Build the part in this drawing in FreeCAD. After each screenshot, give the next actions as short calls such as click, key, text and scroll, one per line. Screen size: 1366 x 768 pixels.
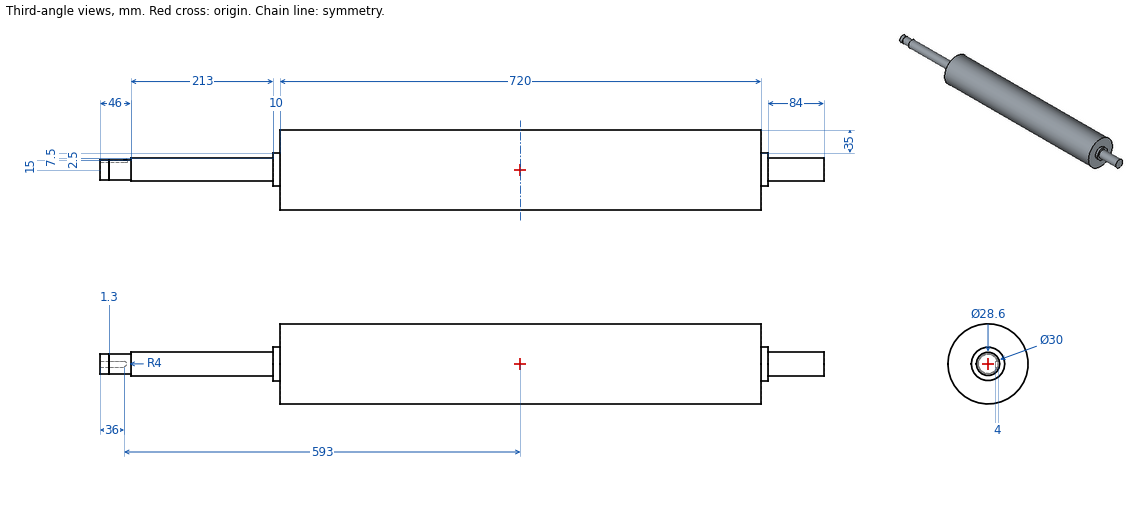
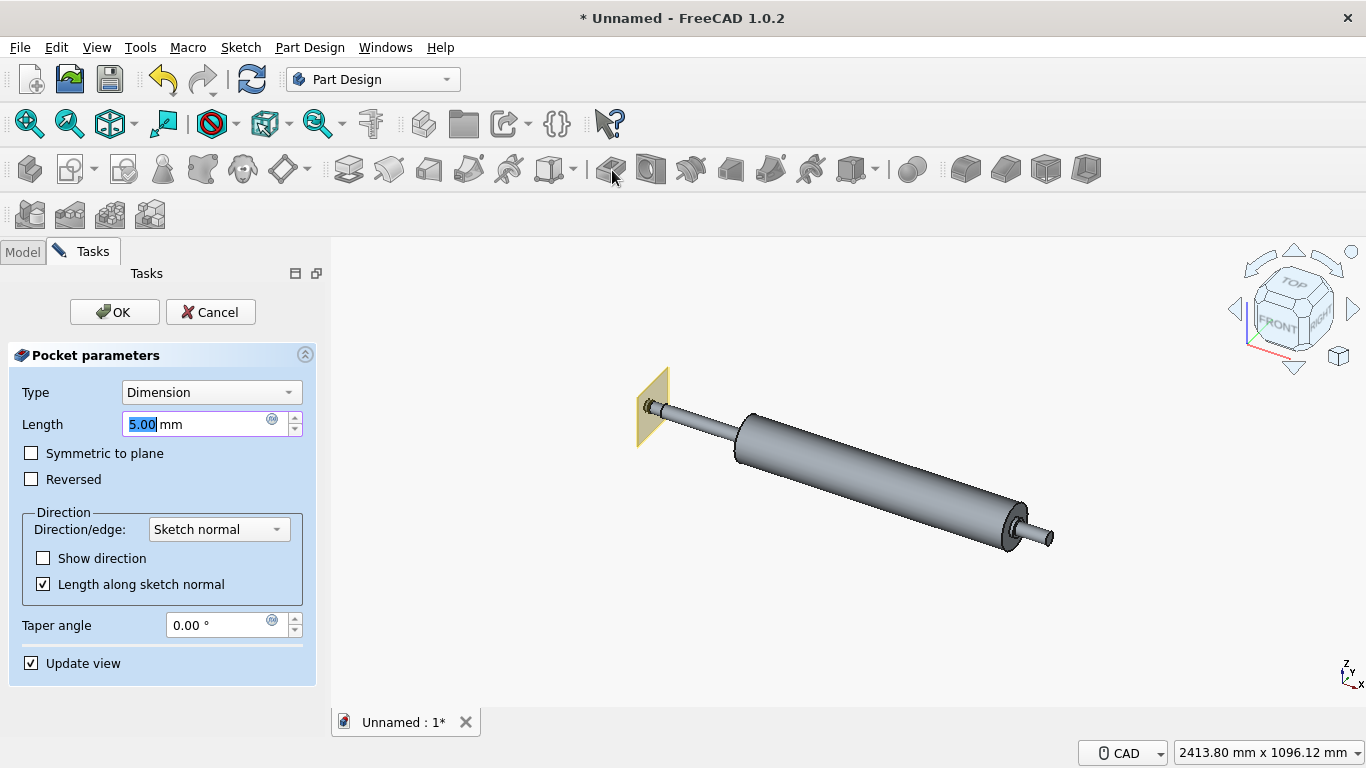
text(1.3)
key(Tab)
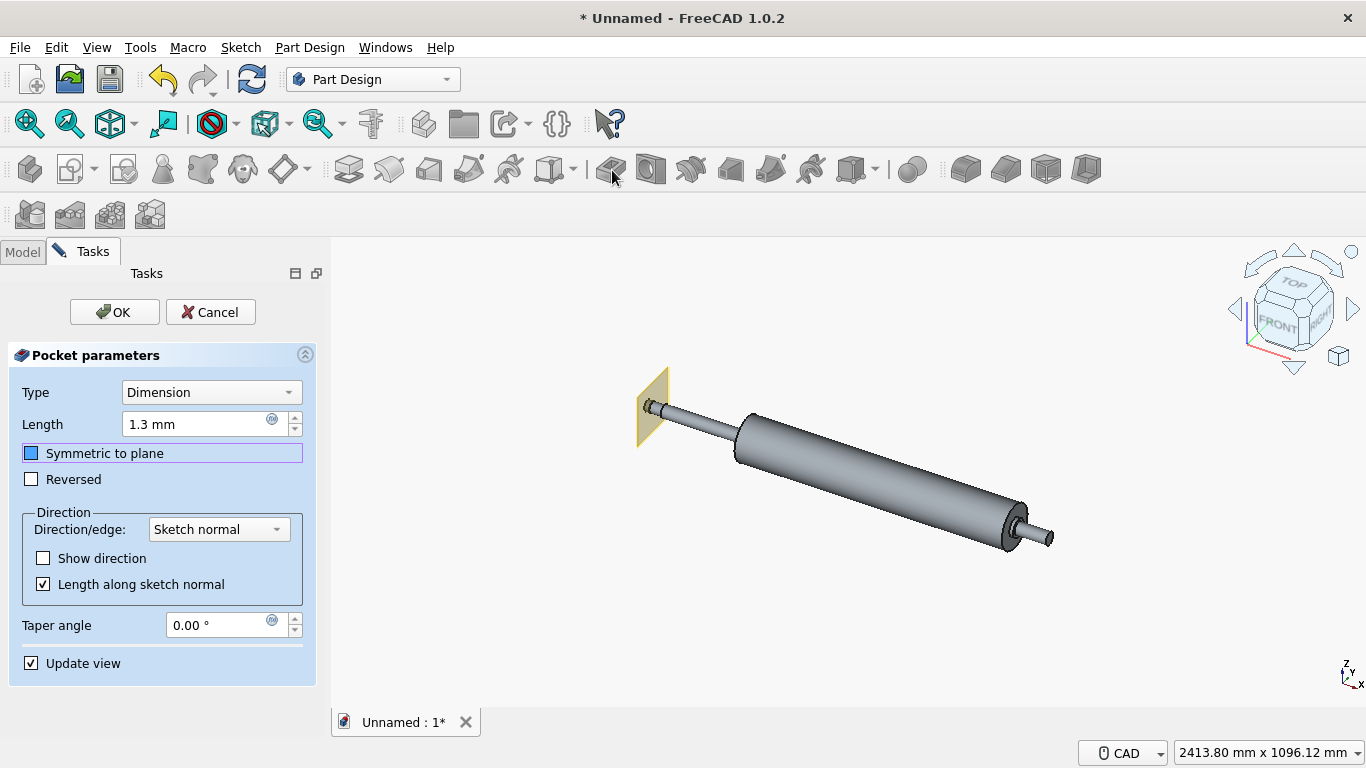
click(115, 312)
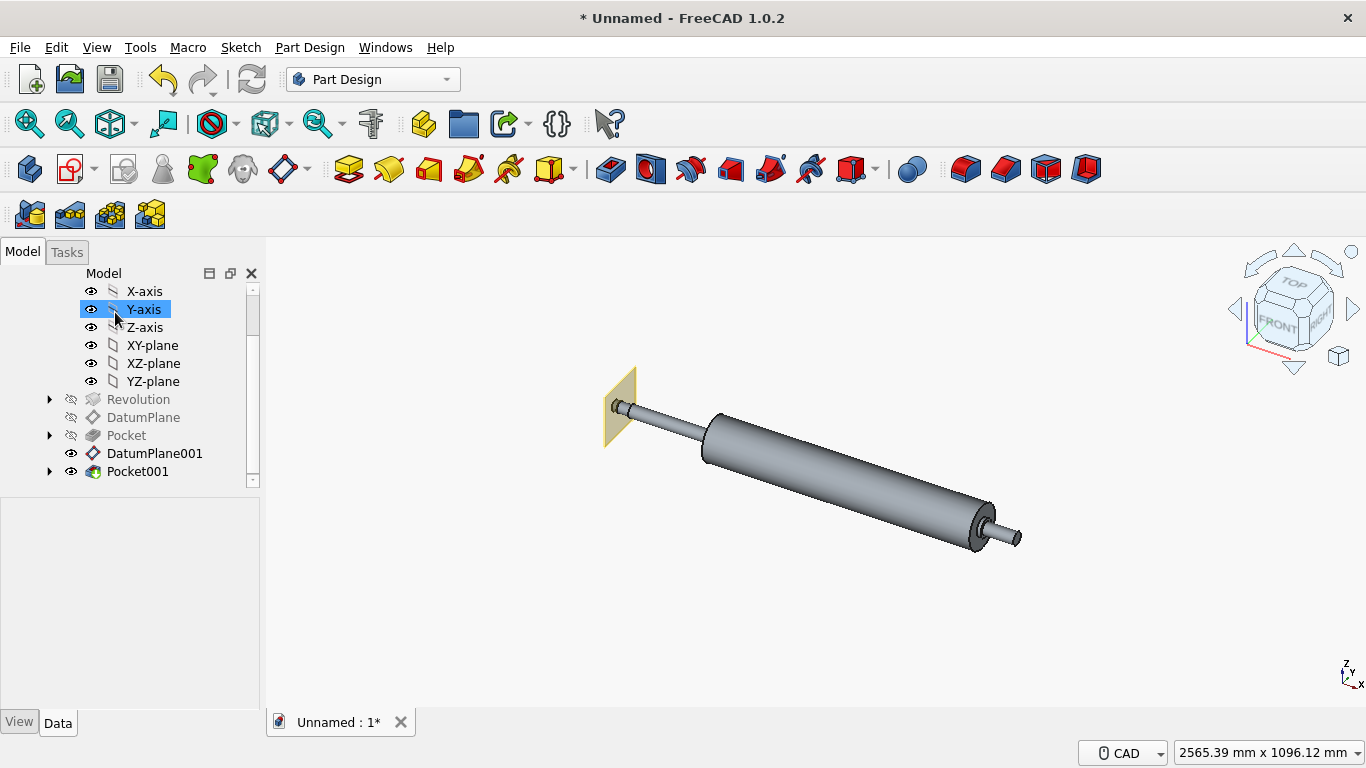
click(116, 453)
key(space)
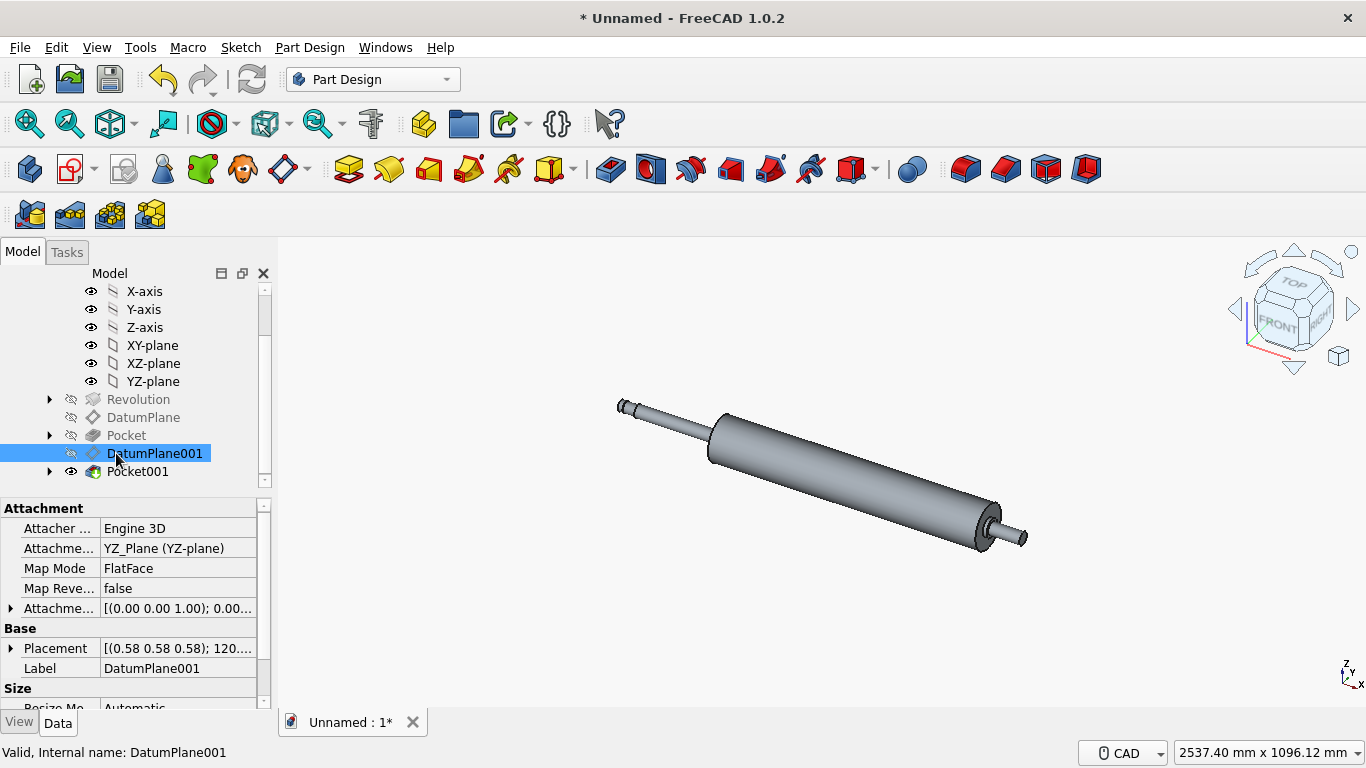
key(0)